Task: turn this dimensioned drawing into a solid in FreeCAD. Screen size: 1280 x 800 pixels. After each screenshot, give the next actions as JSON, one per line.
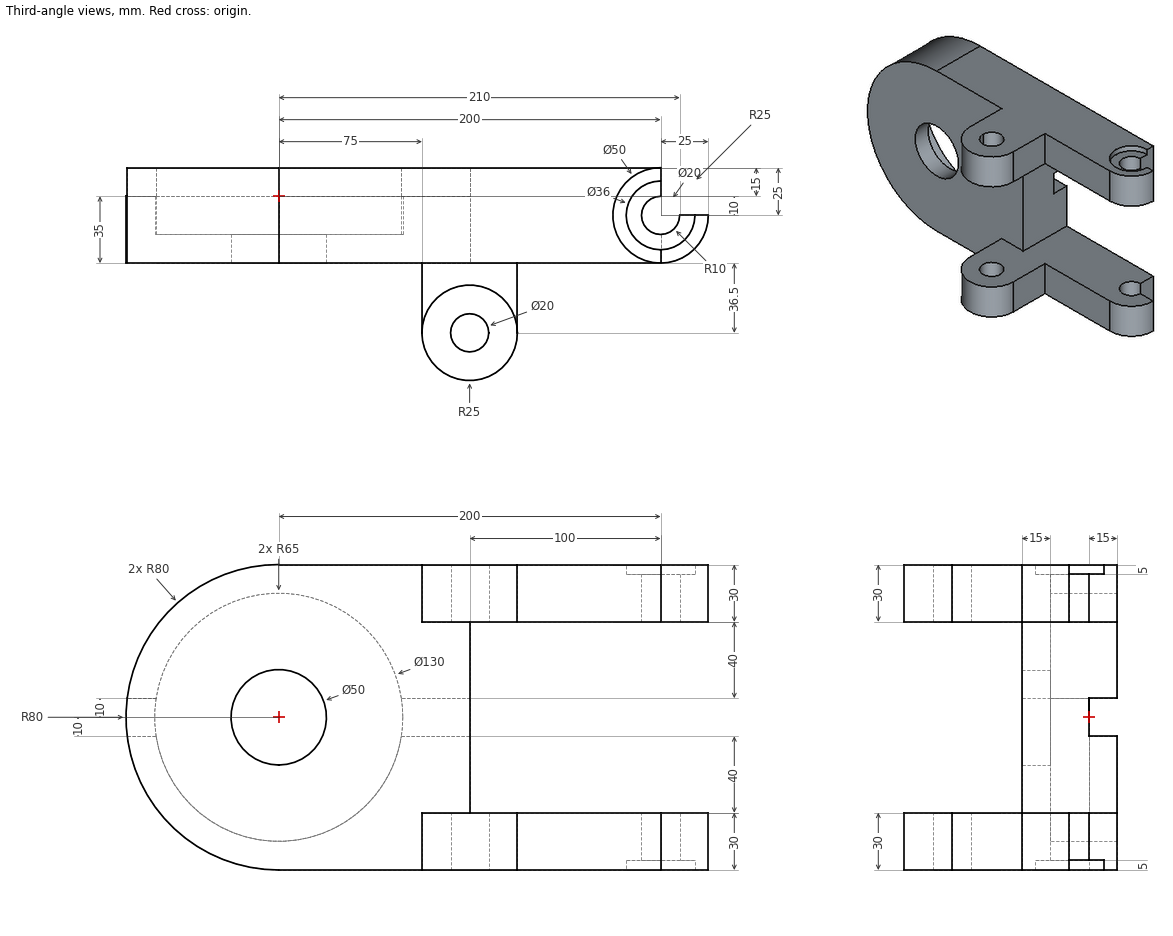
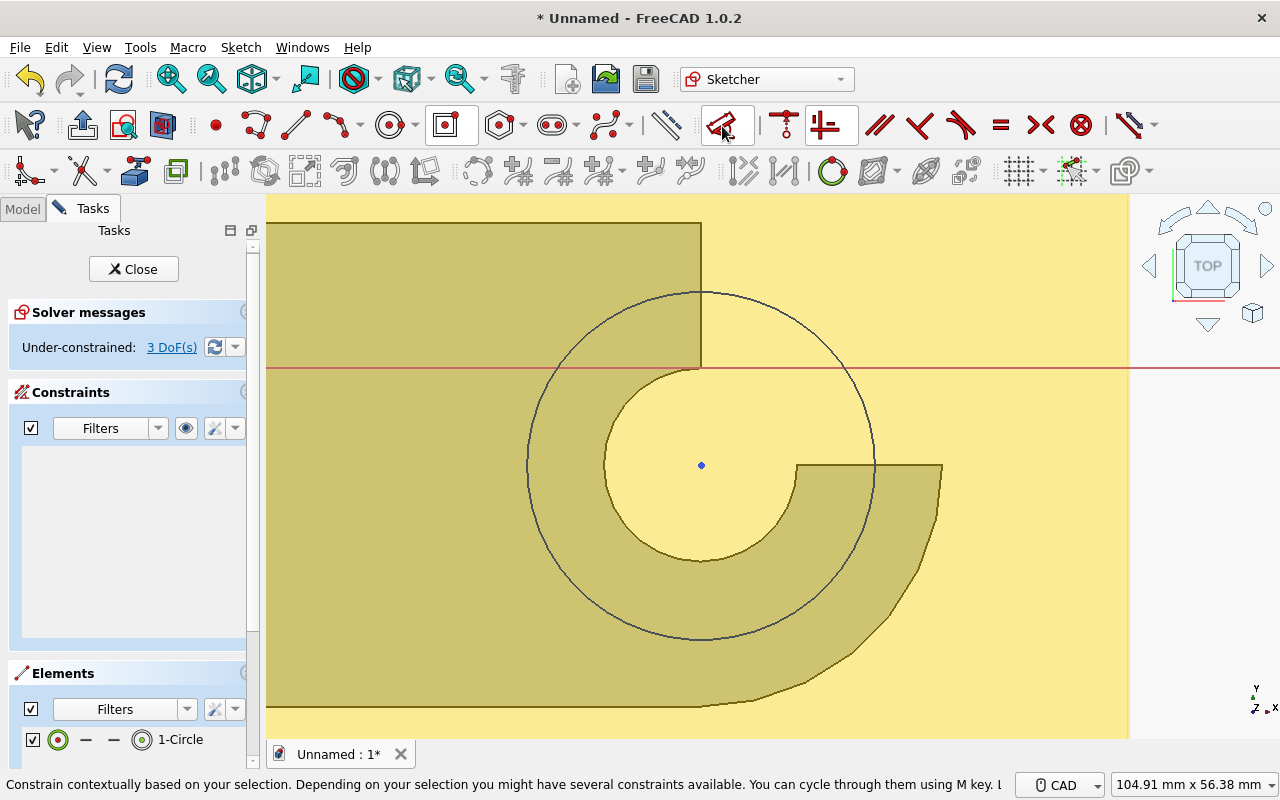
{"action": "left_click", "coordinate": [824, 343]}
{"action": "left_click", "coordinate": [847, 320]}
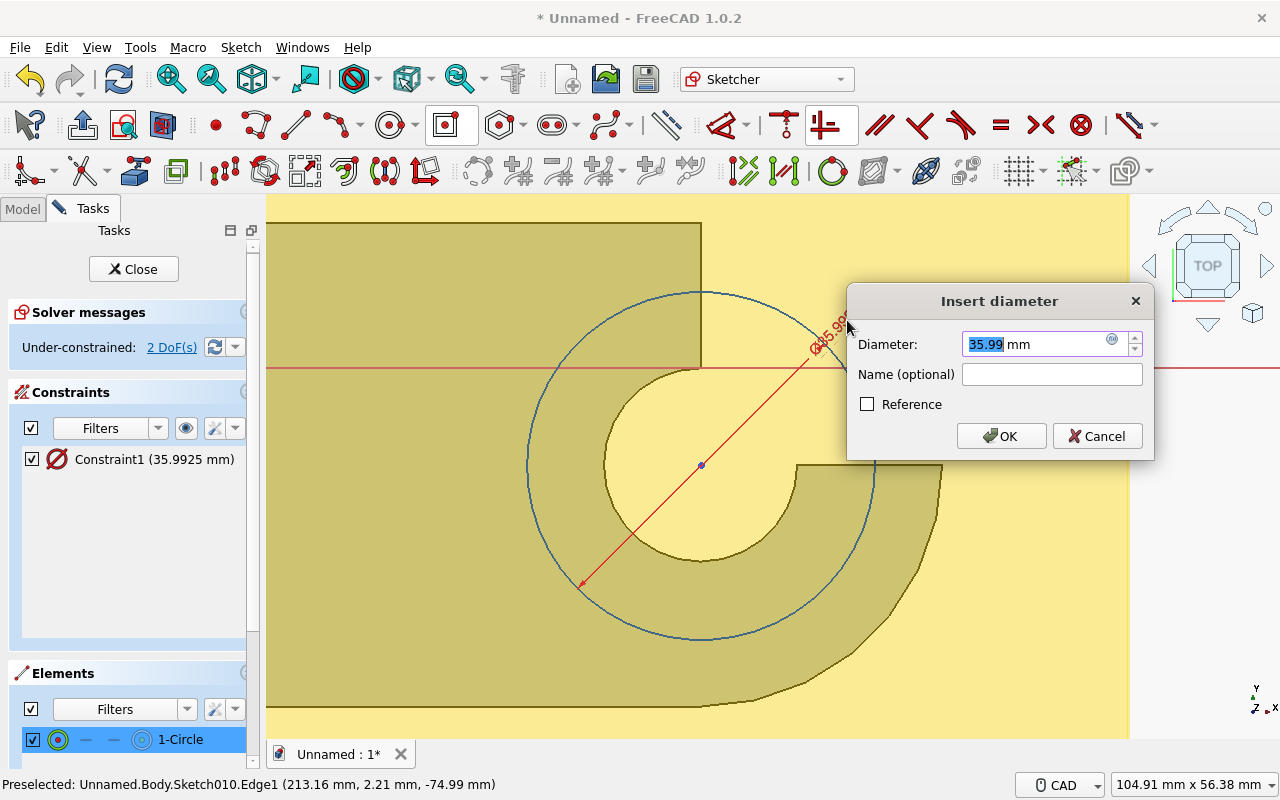
{"action": "type", "text": "36"}
{"action": "key", "text": "Return"}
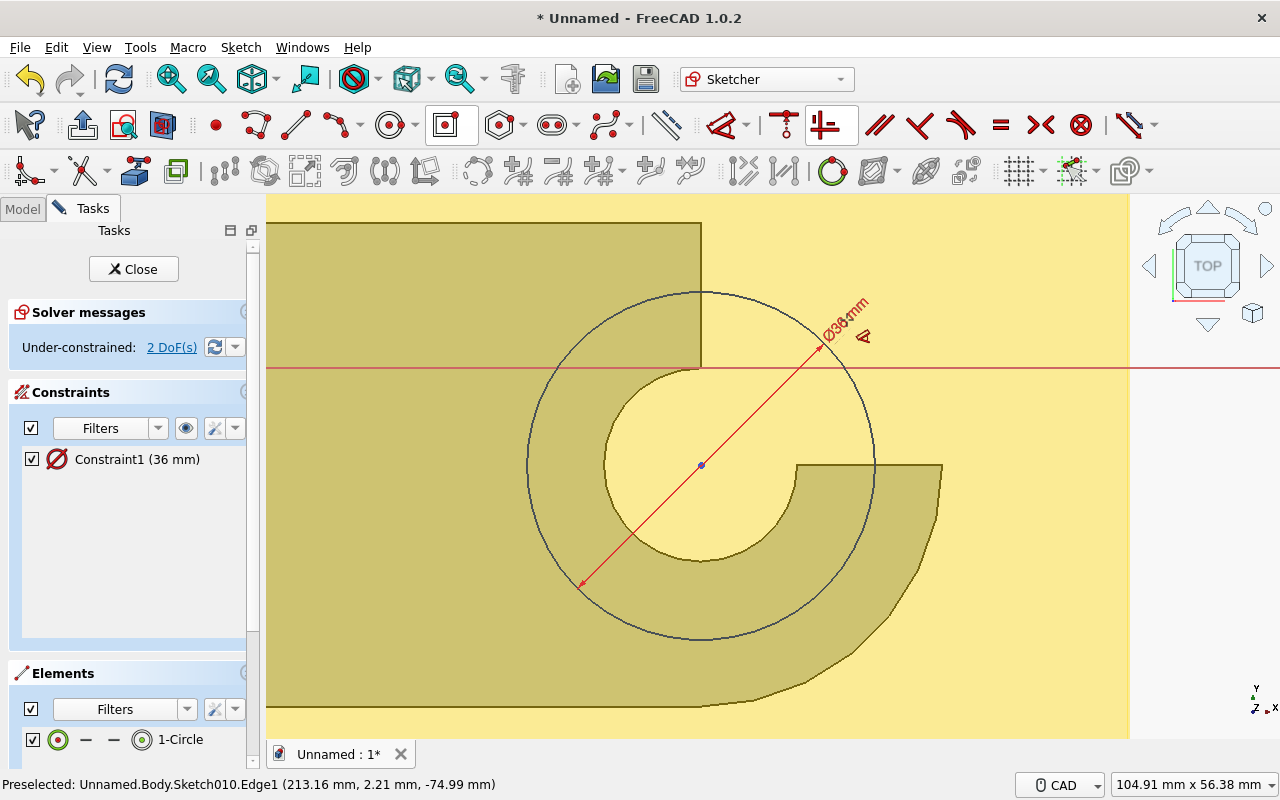
{"action": "left_click", "coordinate": [701, 466]}
{"action": "left_click", "coordinate": [735, 417]}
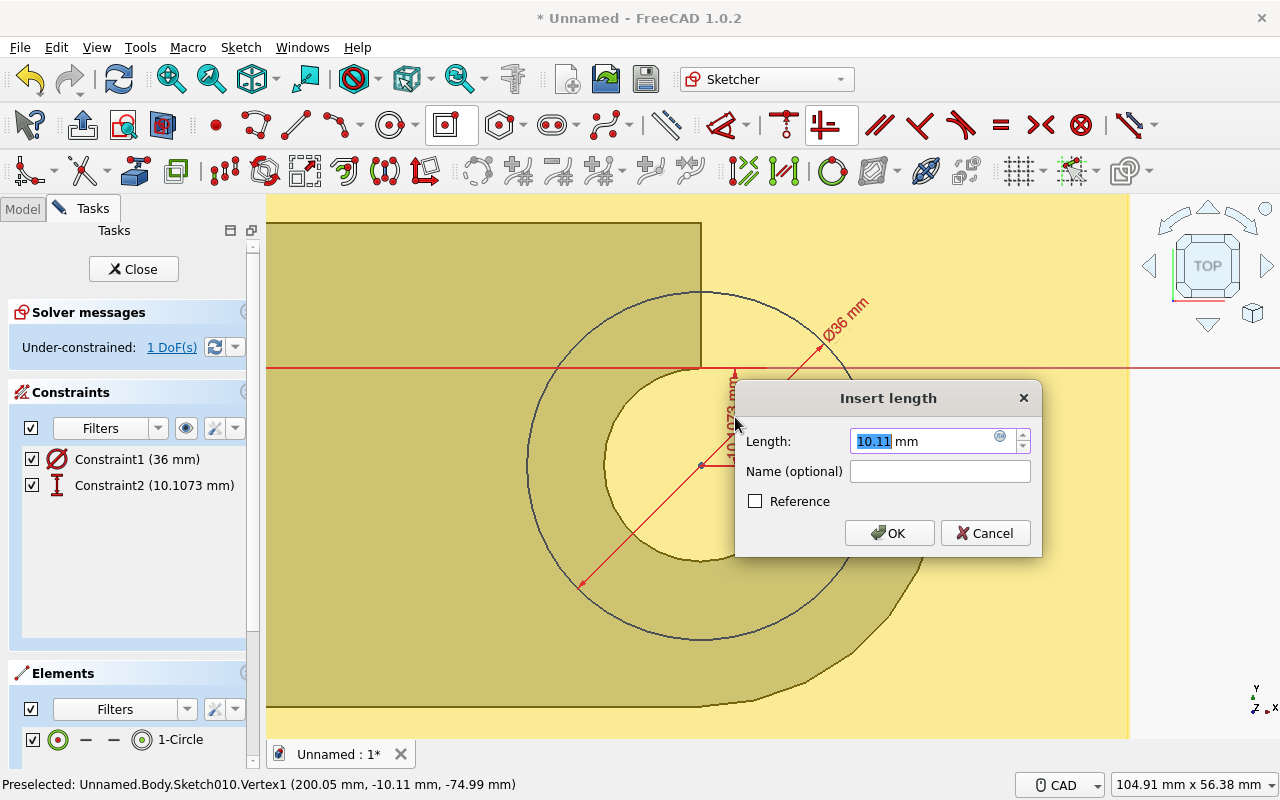
{"action": "type", "text": "10"}
{"action": "key", "text": "Return"}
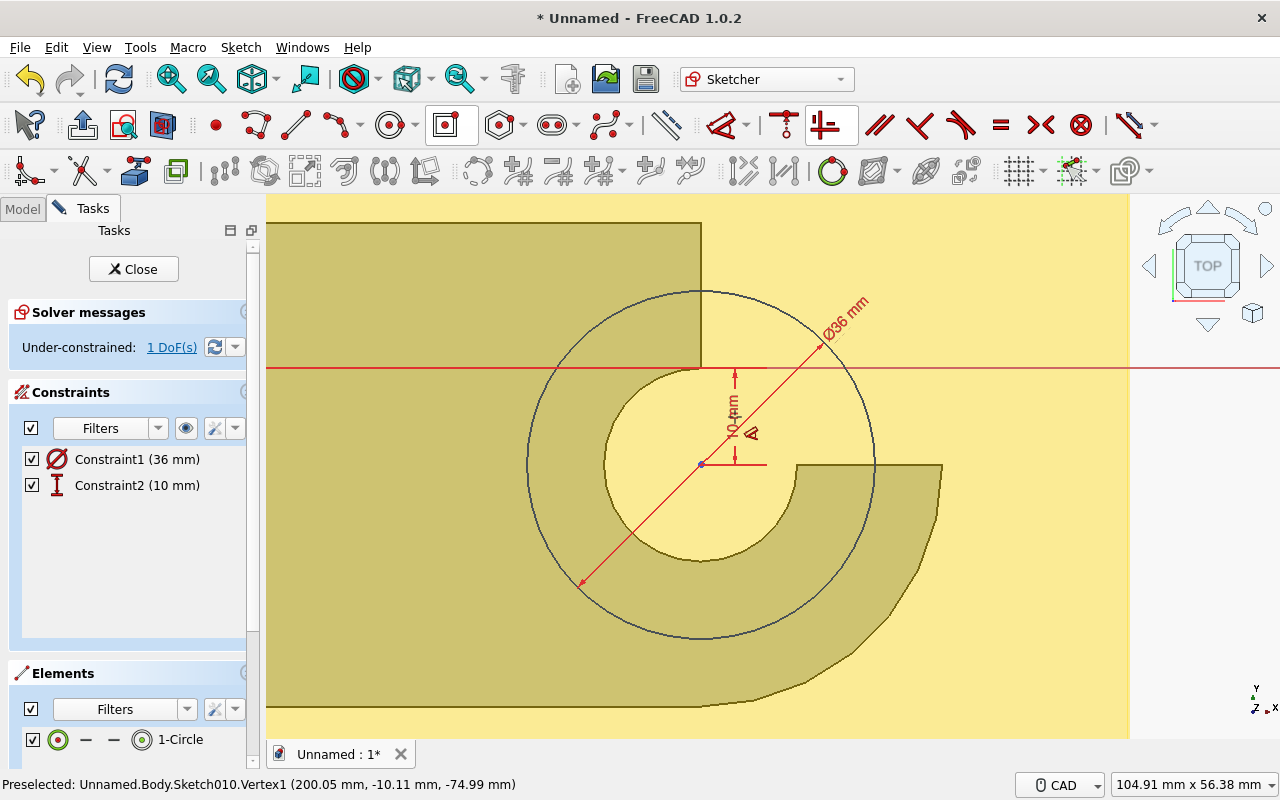
{"action": "left_click", "coordinate": [701, 465]}
{"action": "left_click", "coordinate": [498, 334]}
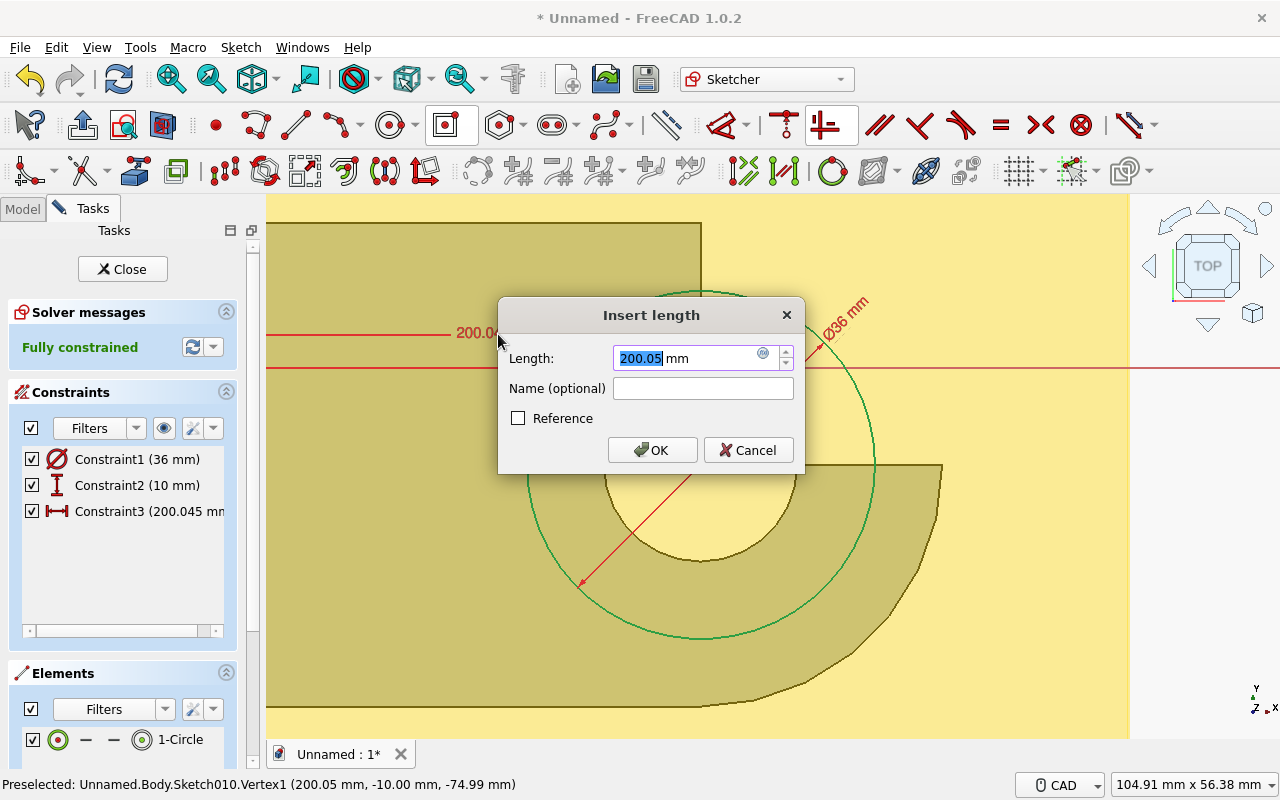
{"action": "type", "text": "200"}
{"action": "key", "text": "Return"}
{"action": "key", "text": "Escape"}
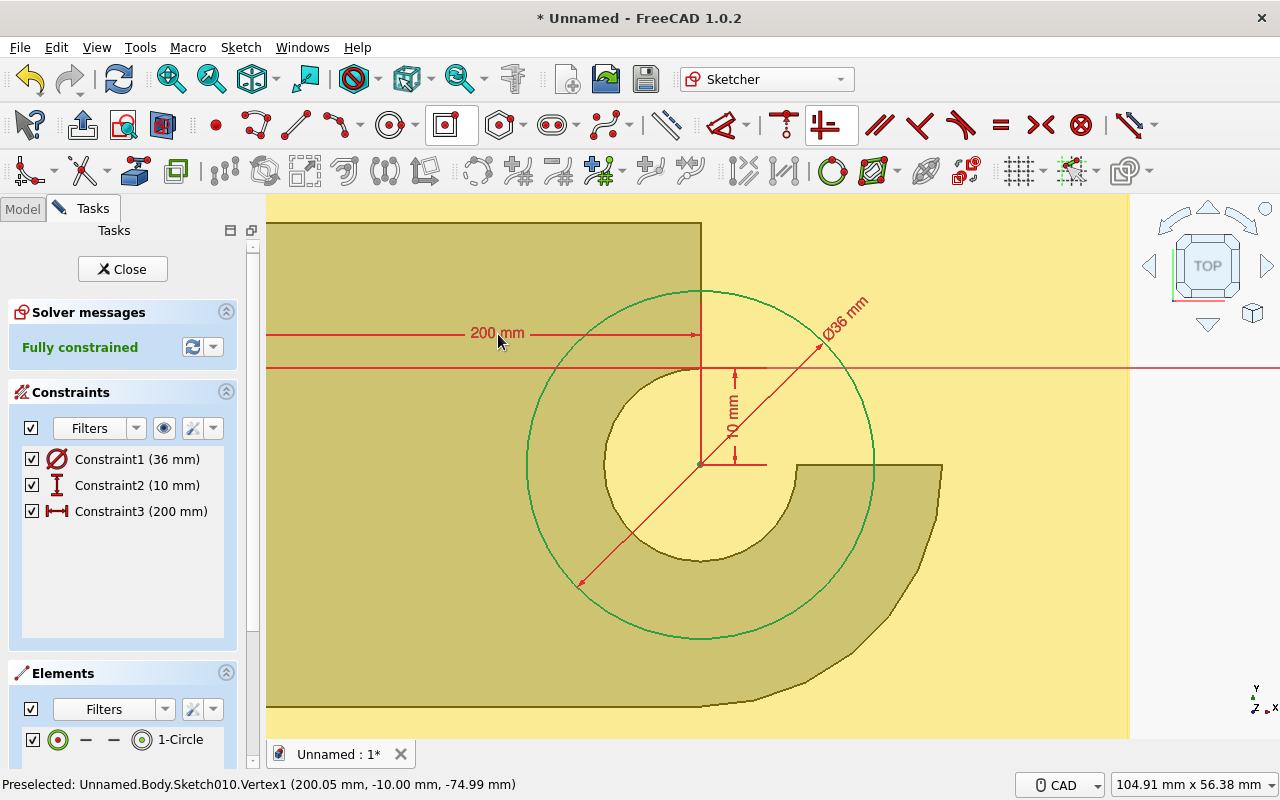
{"action": "left_click", "coordinate": [123, 269]}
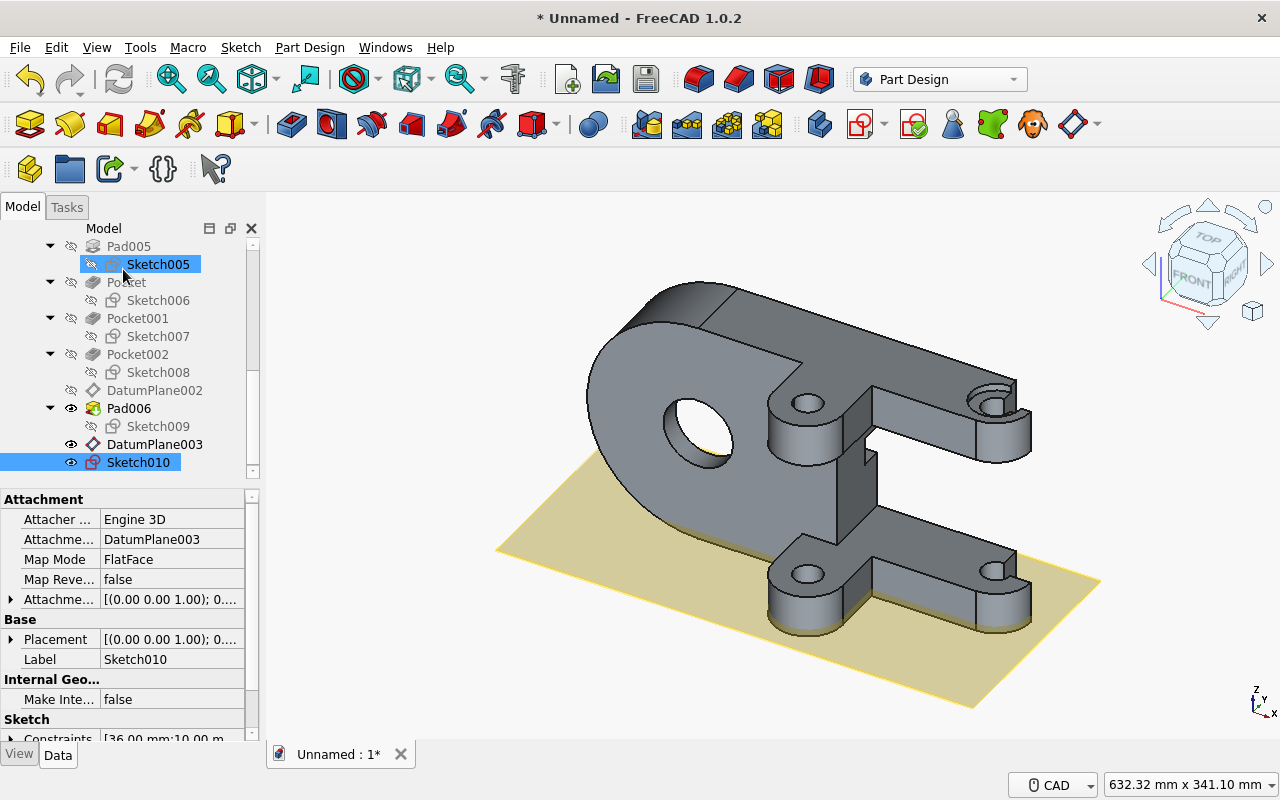
{"action": "left_click", "coordinate": [292, 124]}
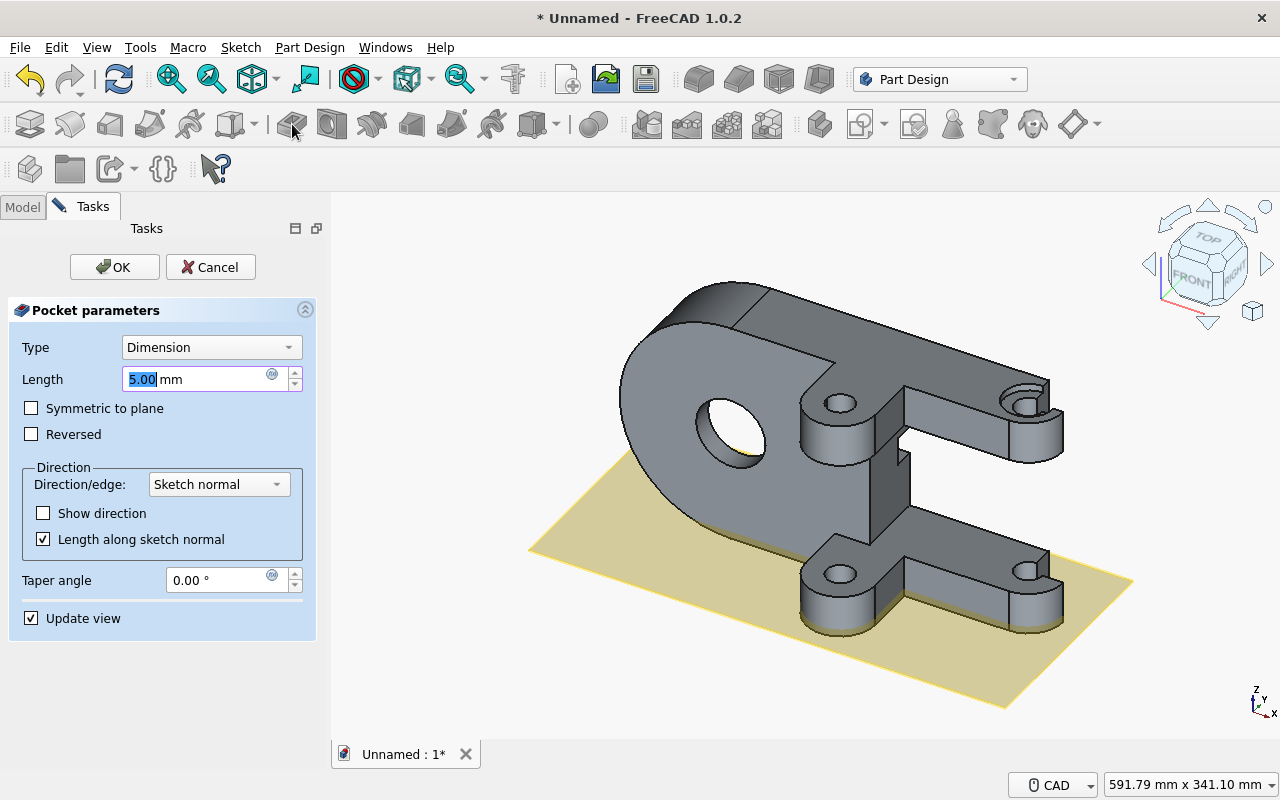
{"action": "type", "text": "5"}
{"action": "key", "text": "Tab"}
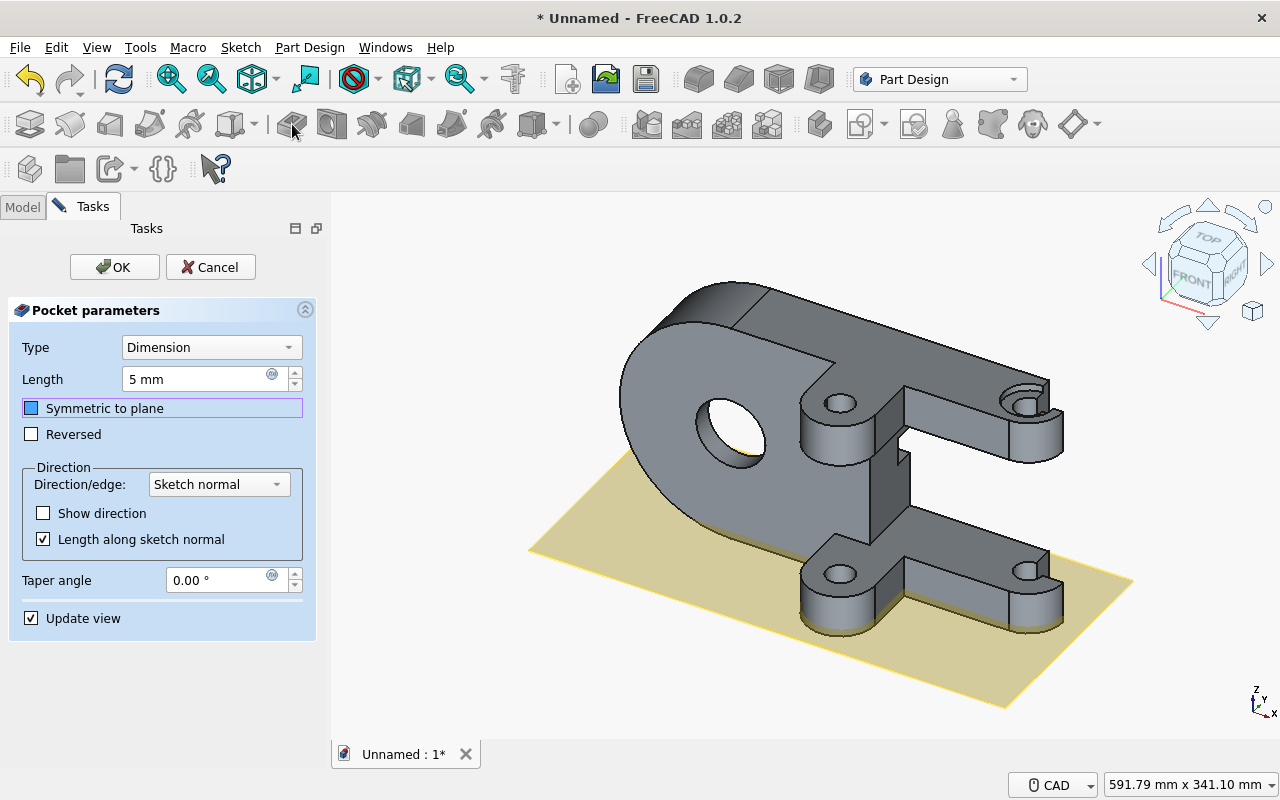
{"action": "left_click", "coordinate": [115, 267]}